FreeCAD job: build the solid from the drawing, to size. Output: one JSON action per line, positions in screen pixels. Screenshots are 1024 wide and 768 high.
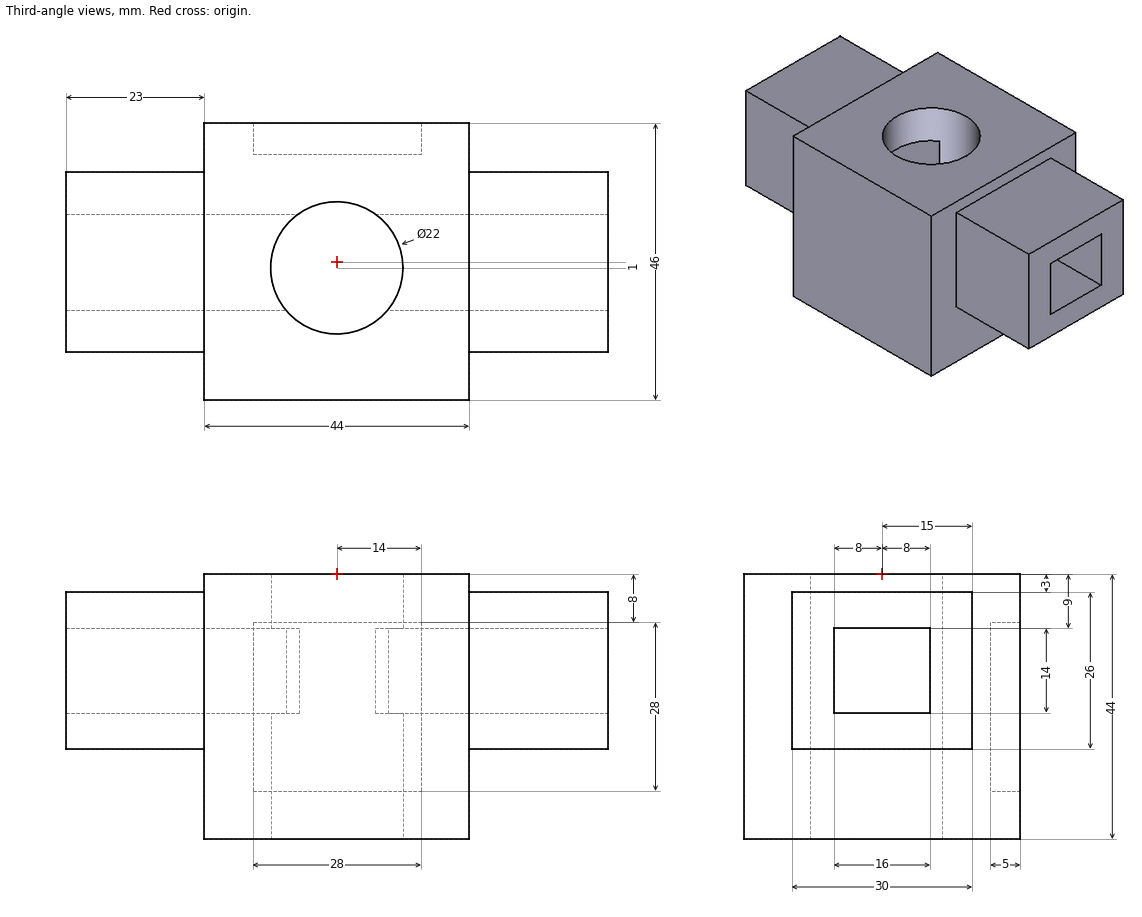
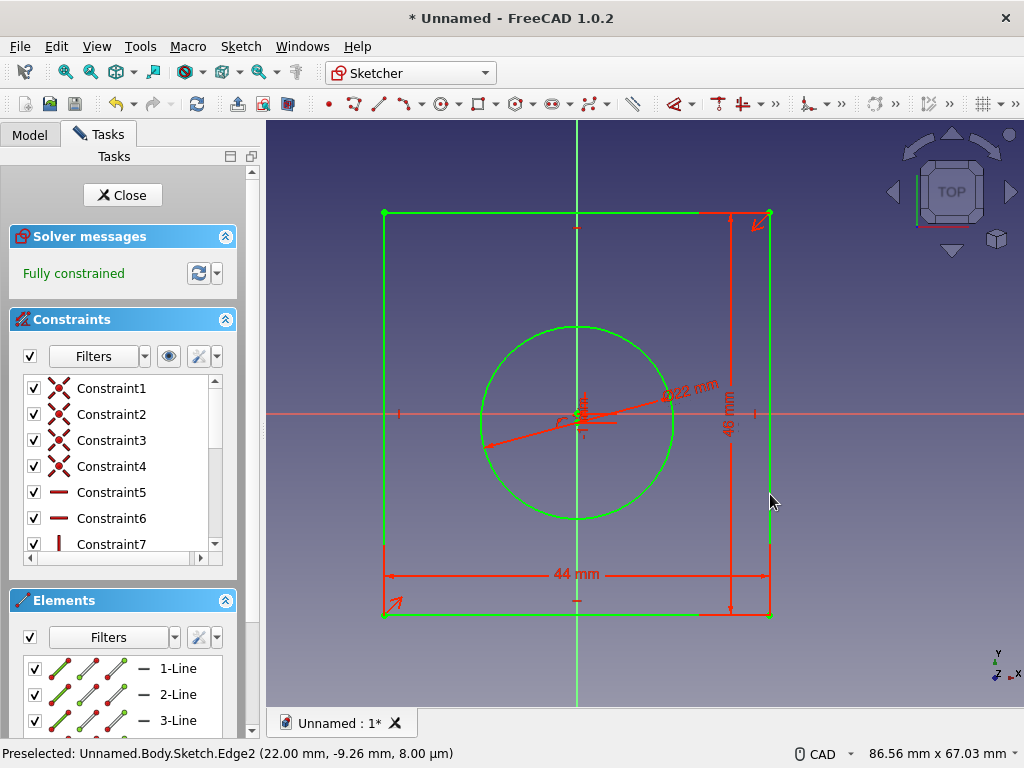
{"action": "left_click", "coordinate": [123, 195]}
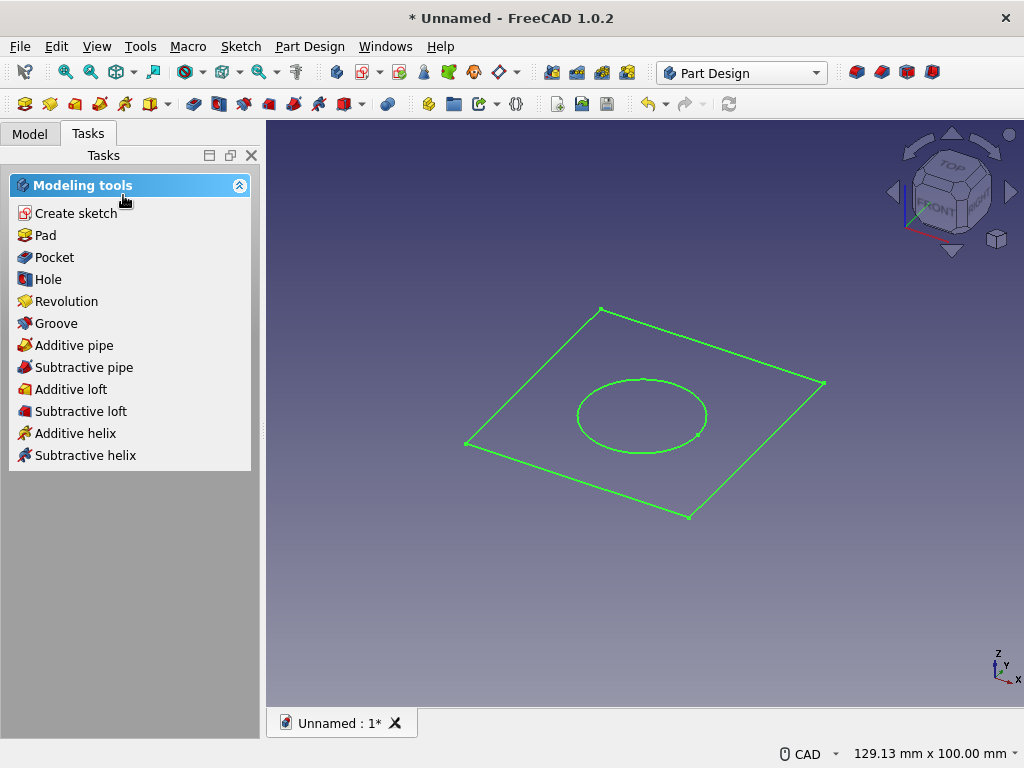
{"action": "left_click", "coordinate": [25, 104]}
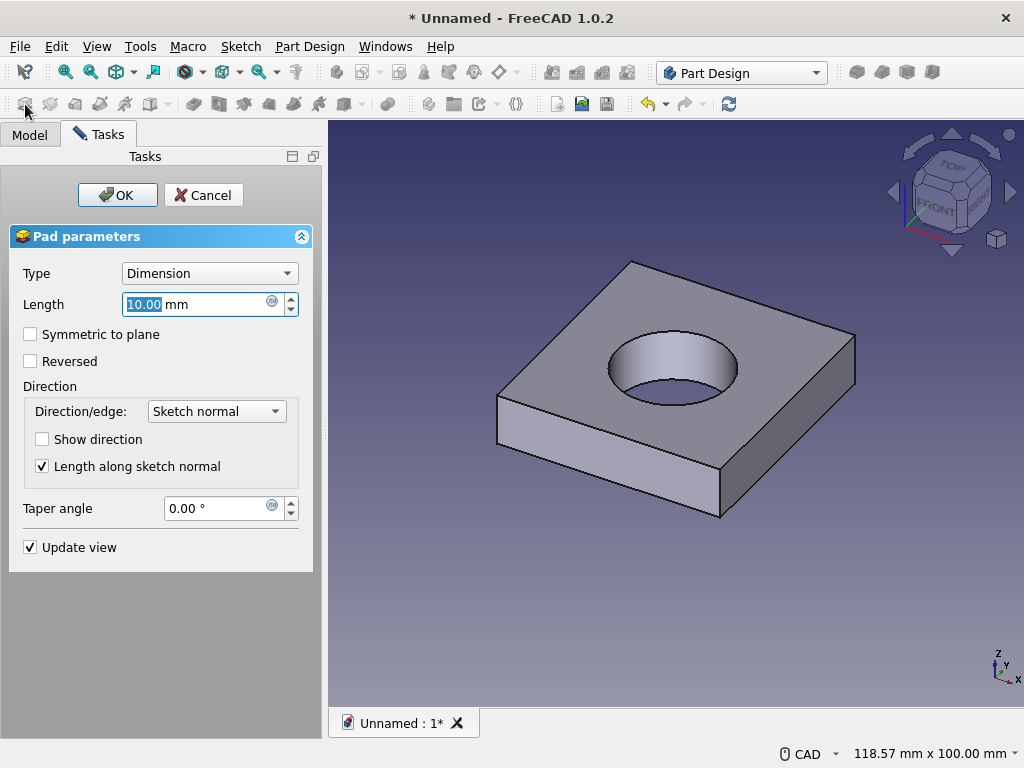
{"action": "type", "text": "44"}
{"action": "key", "text": "Tab"}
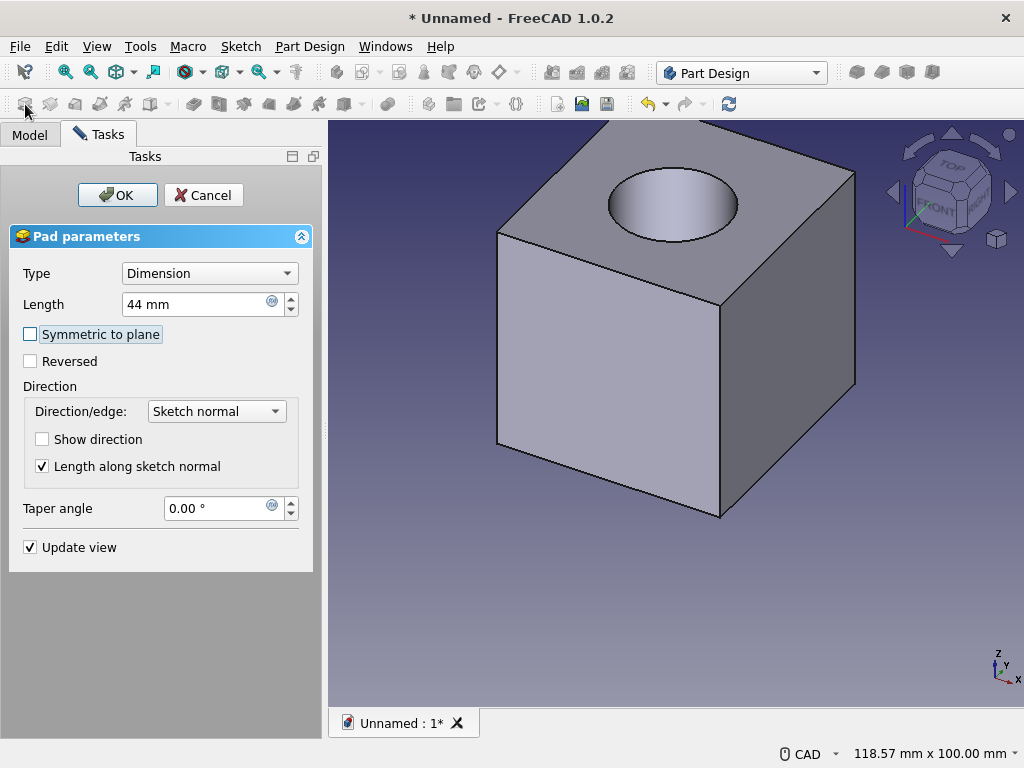
{"action": "left_click", "coordinate": [31, 361]}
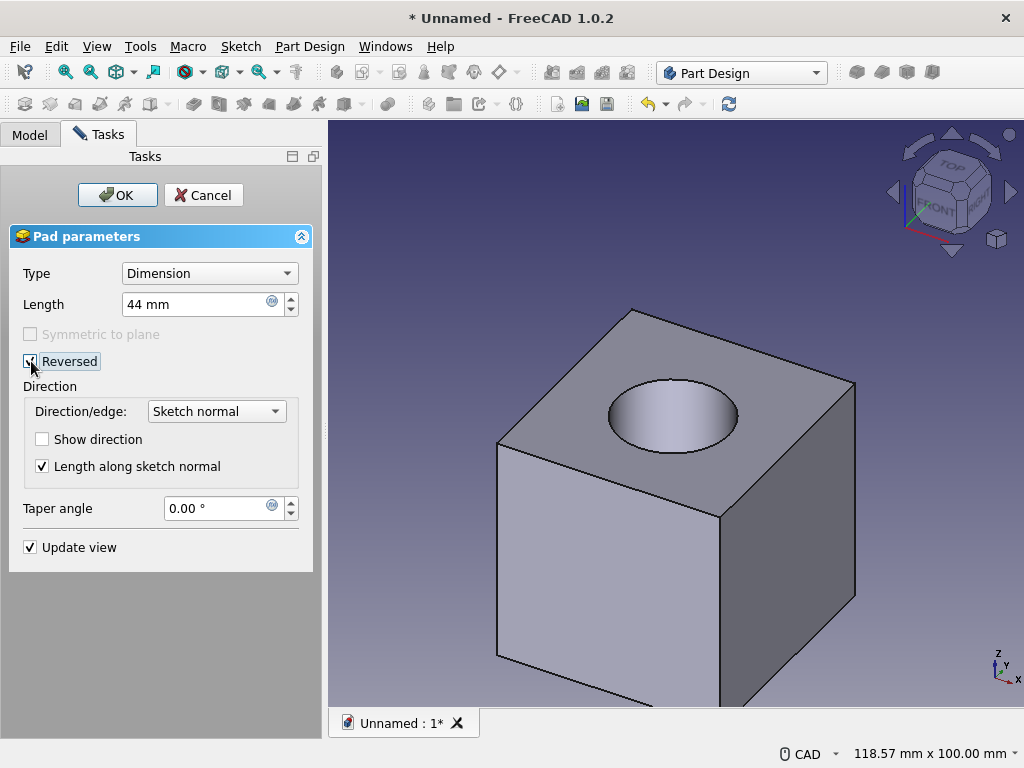
{"action": "left_click", "coordinate": [118, 195]}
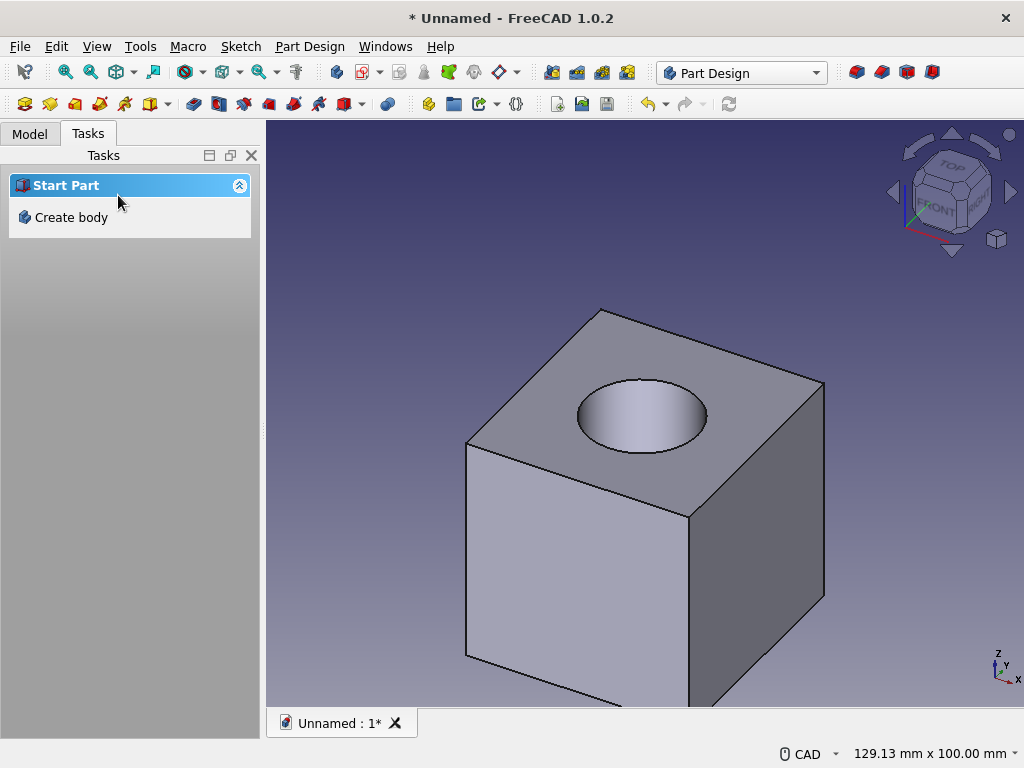
{"action": "left_click", "coordinate": [66, 72]}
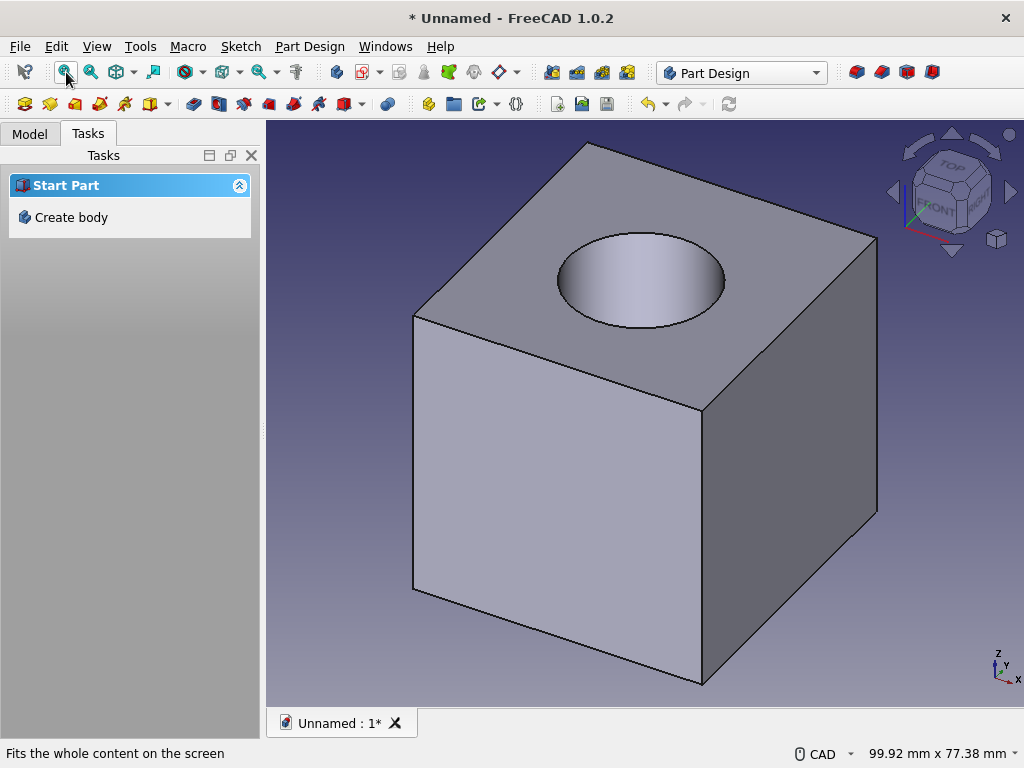
{"action": "key", "text": "4"}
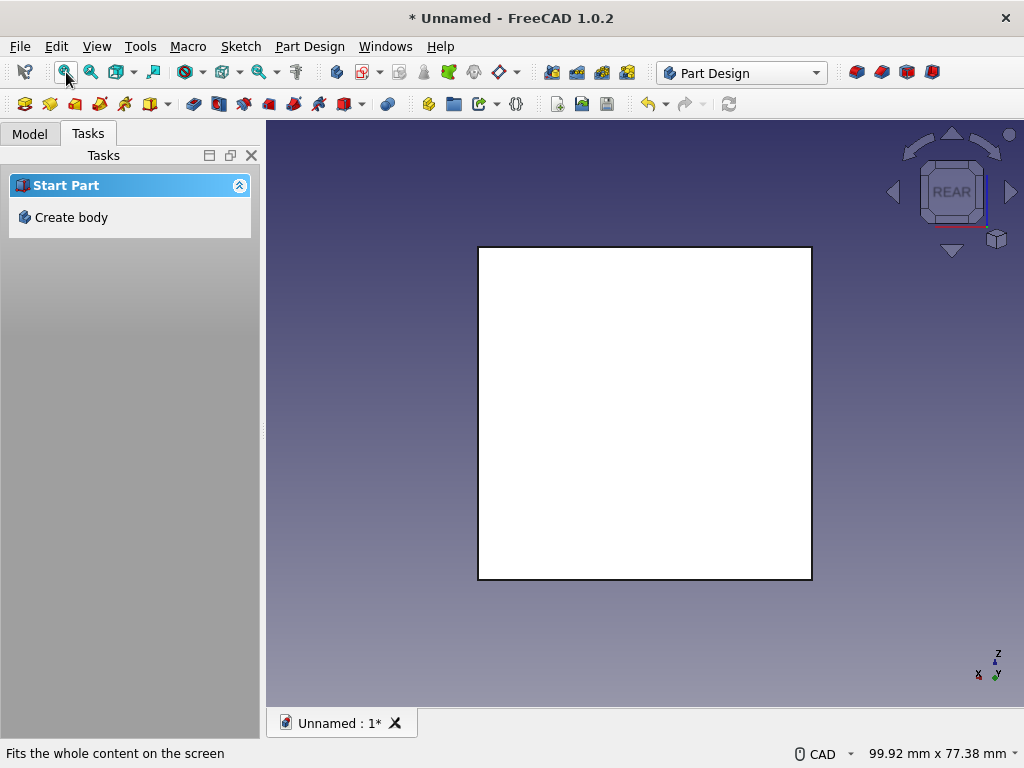
{"action": "left_click", "coordinate": [645, 412]}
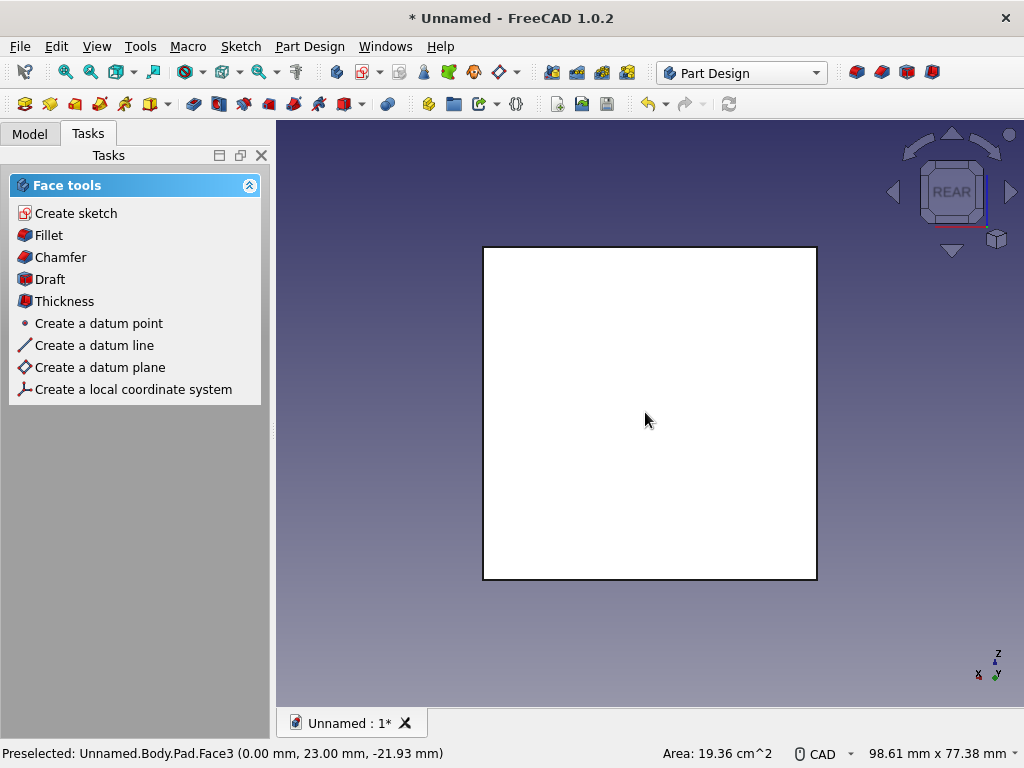
{"action": "left_click", "coordinate": [362, 72]}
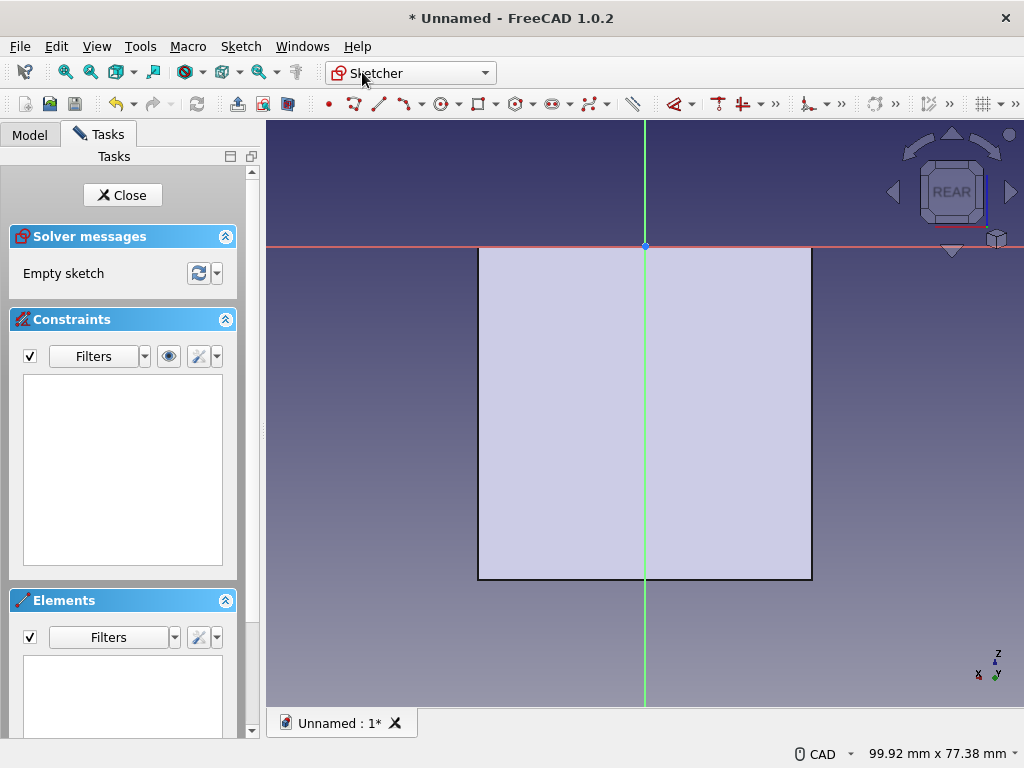
{"action": "scroll", "coordinate": [784, 321], "scroll_direction": "up", "scroll_amount": 2}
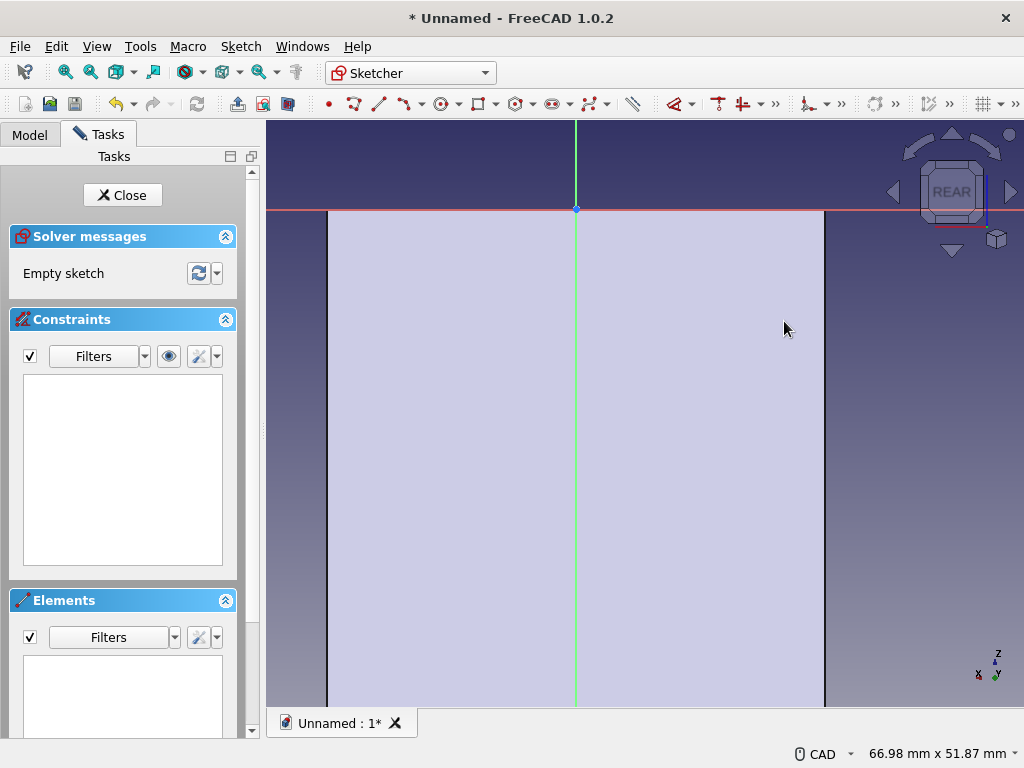
{"action": "key", "text": "g r"}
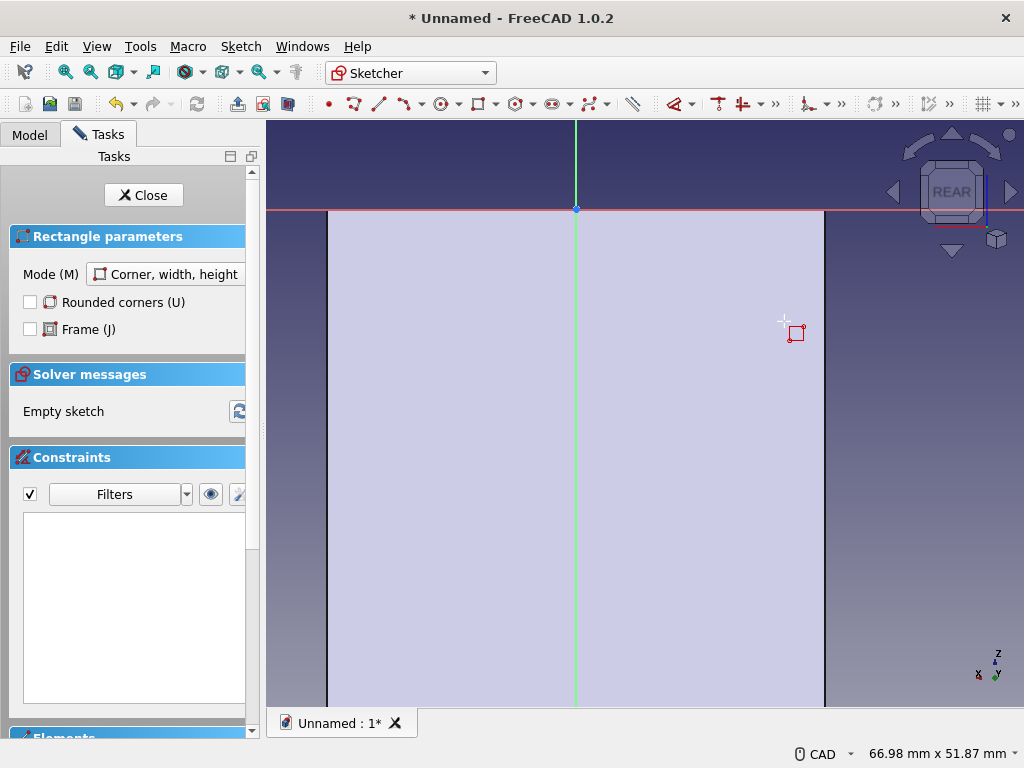
{"action": "left_click", "coordinate": [418, 300]}
{"action": "left_click", "coordinate": [735, 617]}
{"action": "key", "text": "Escape"}